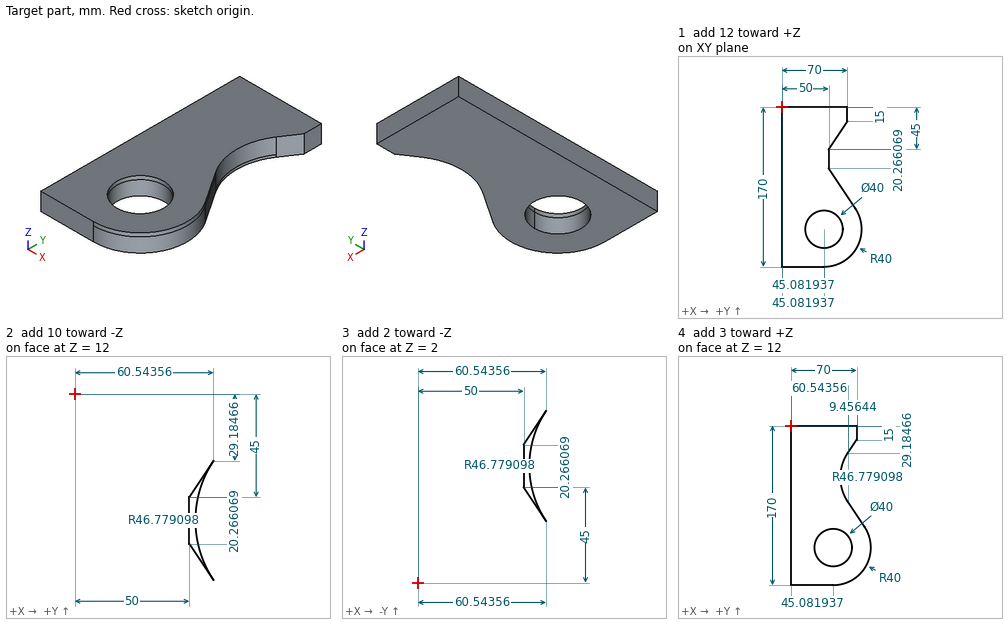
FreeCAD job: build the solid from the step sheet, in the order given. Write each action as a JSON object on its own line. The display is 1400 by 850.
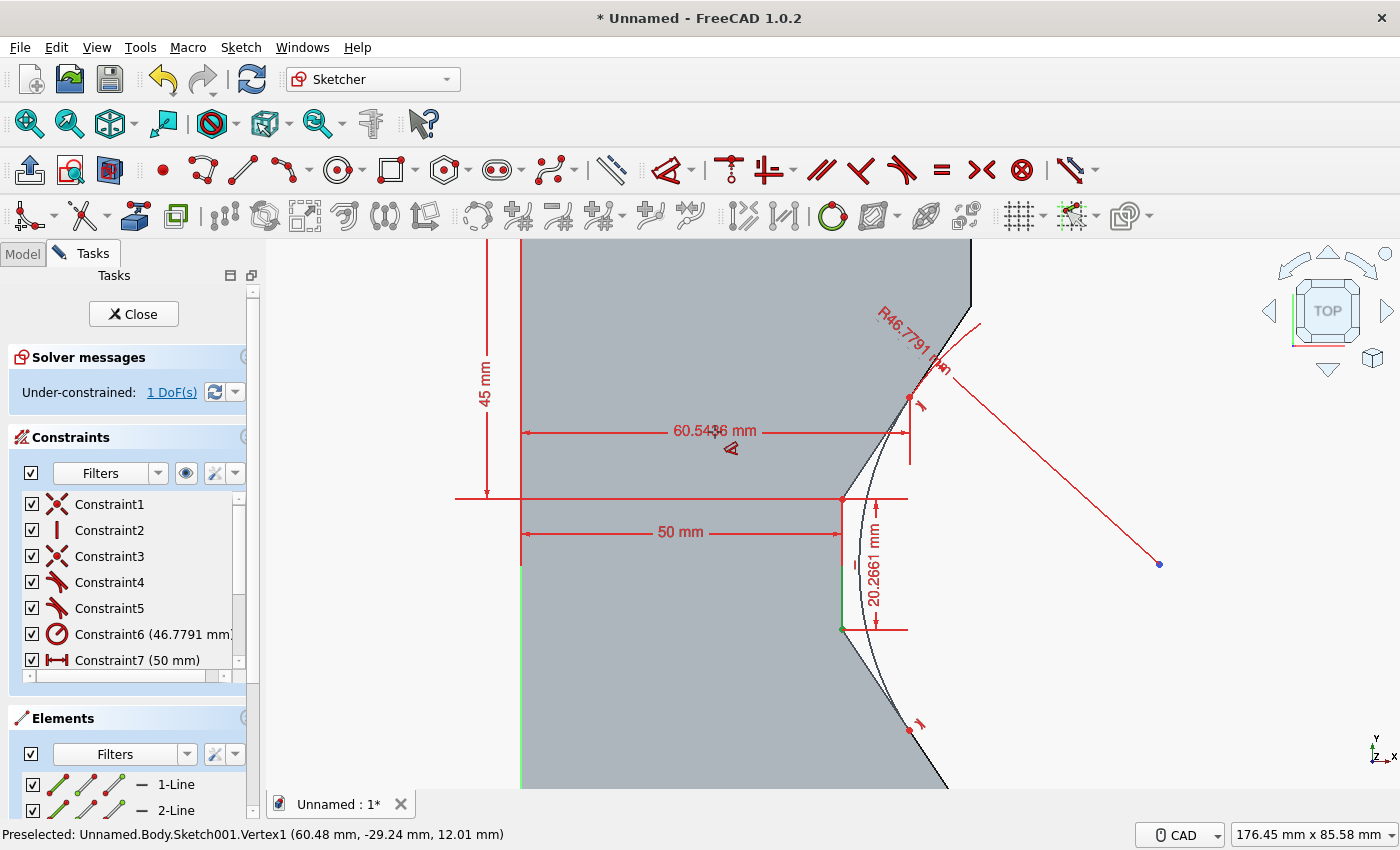
{"action": "left_click", "coordinate": [910, 398]}
{"action": "left_click", "coordinate": [487, 332]}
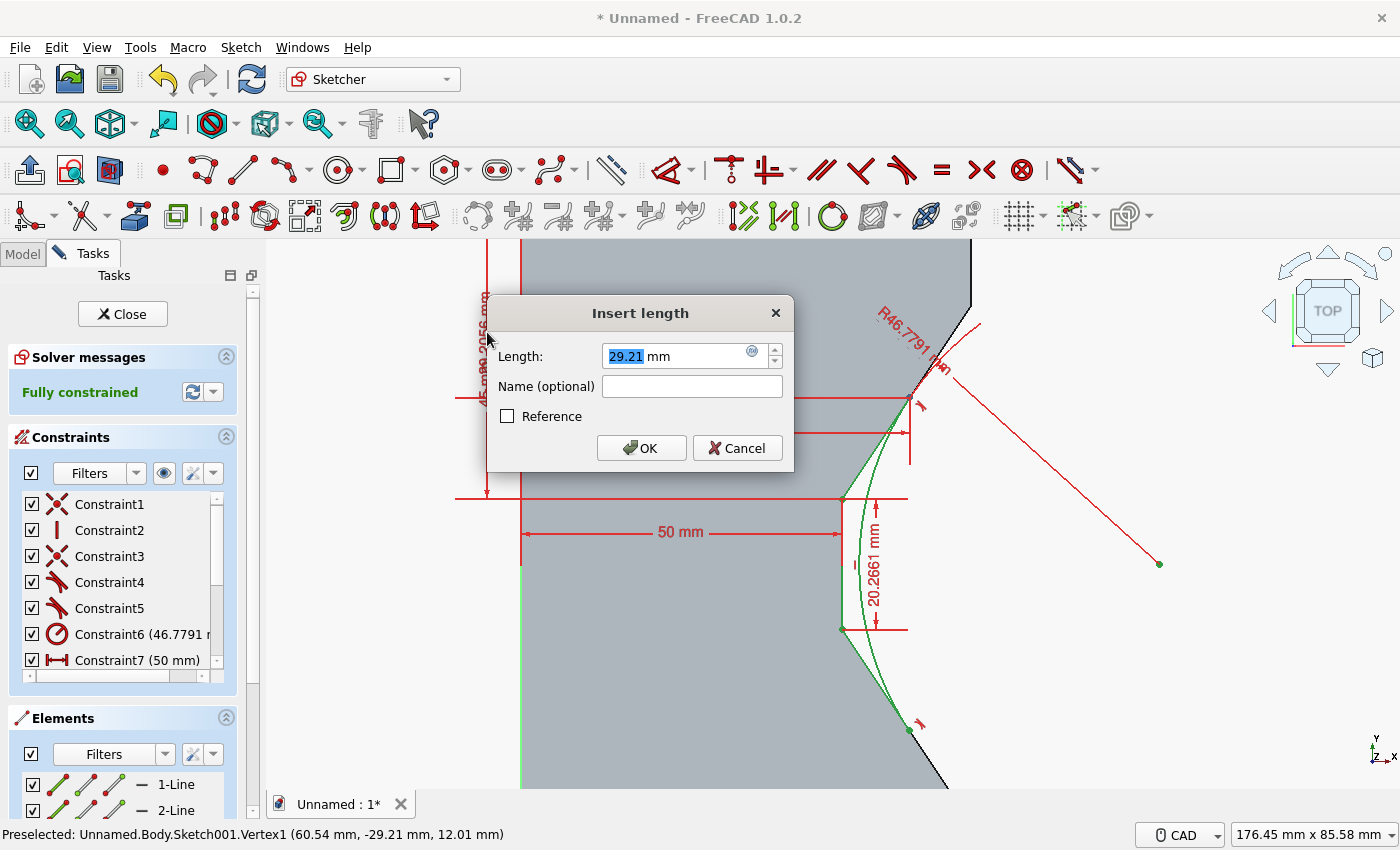
{"action": "type", "text": "29.18466"}
{"action": "key", "text": "Return"}
{"action": "key", "text": "Escape"}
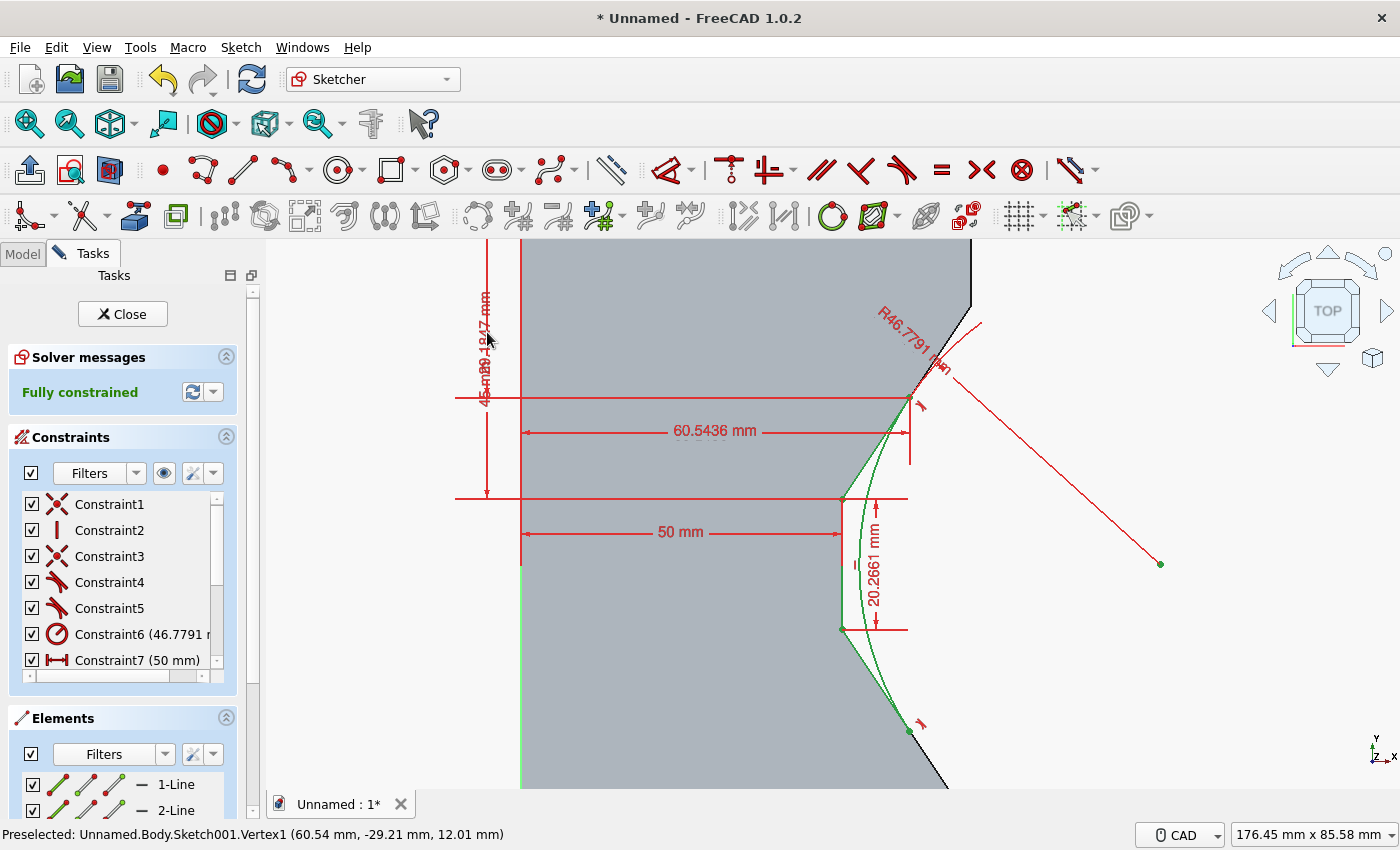
{"action": "left_click", "coordinate": [123, 314]}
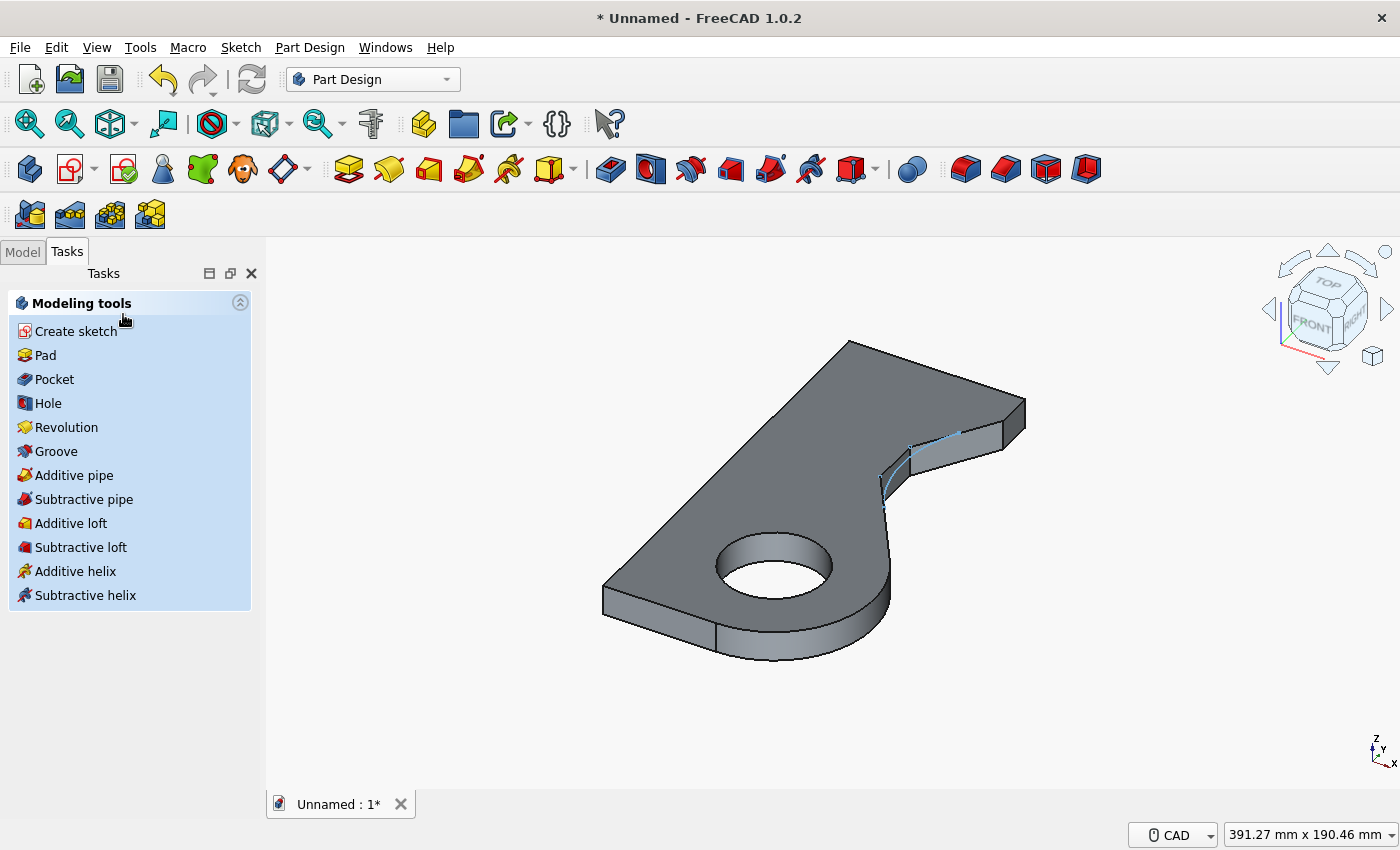
{"action": "left_click", "coordinate": [350, 170]}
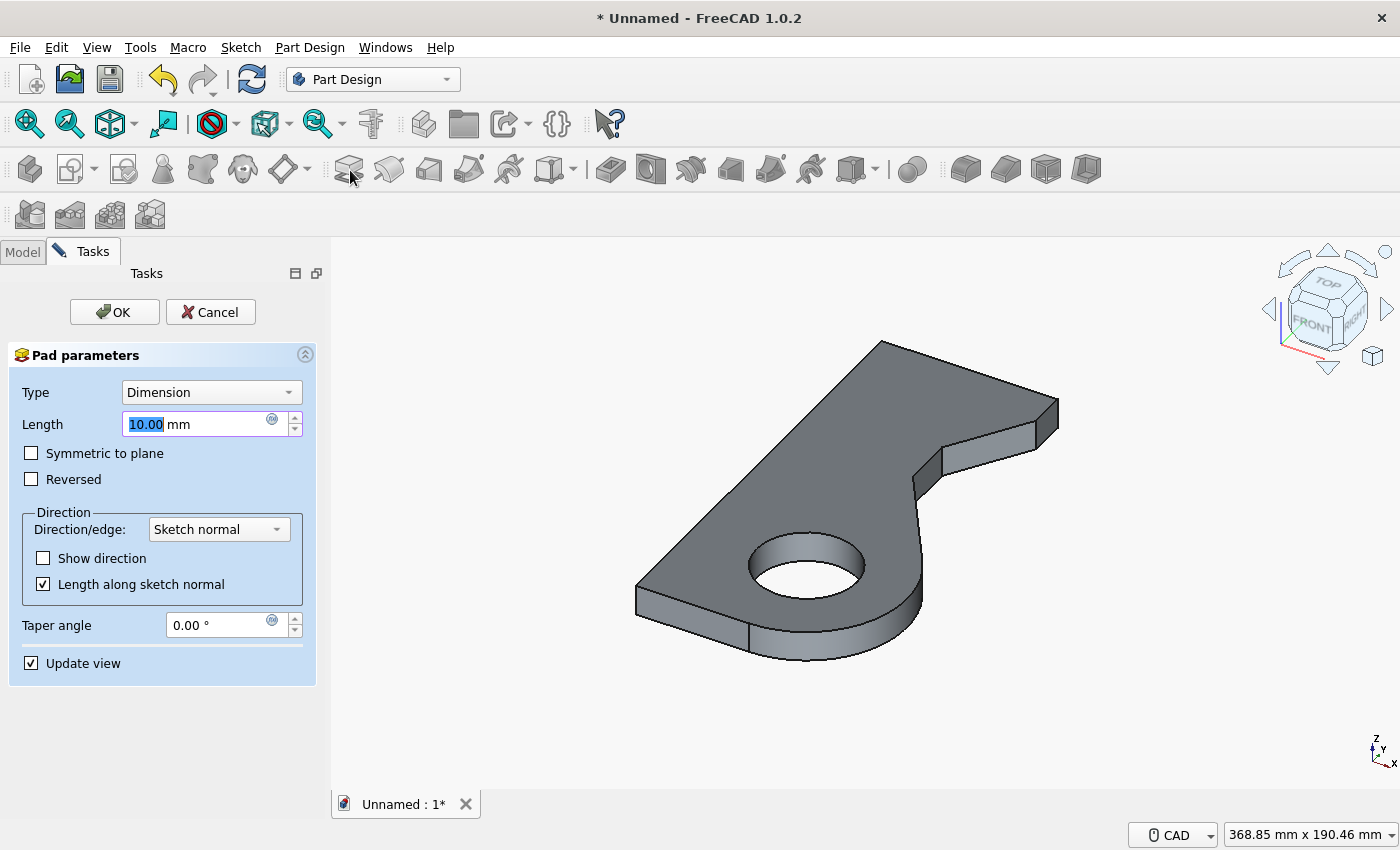
{"action": "type", "text": "10"}
{"action": "key", "text": "Tab"}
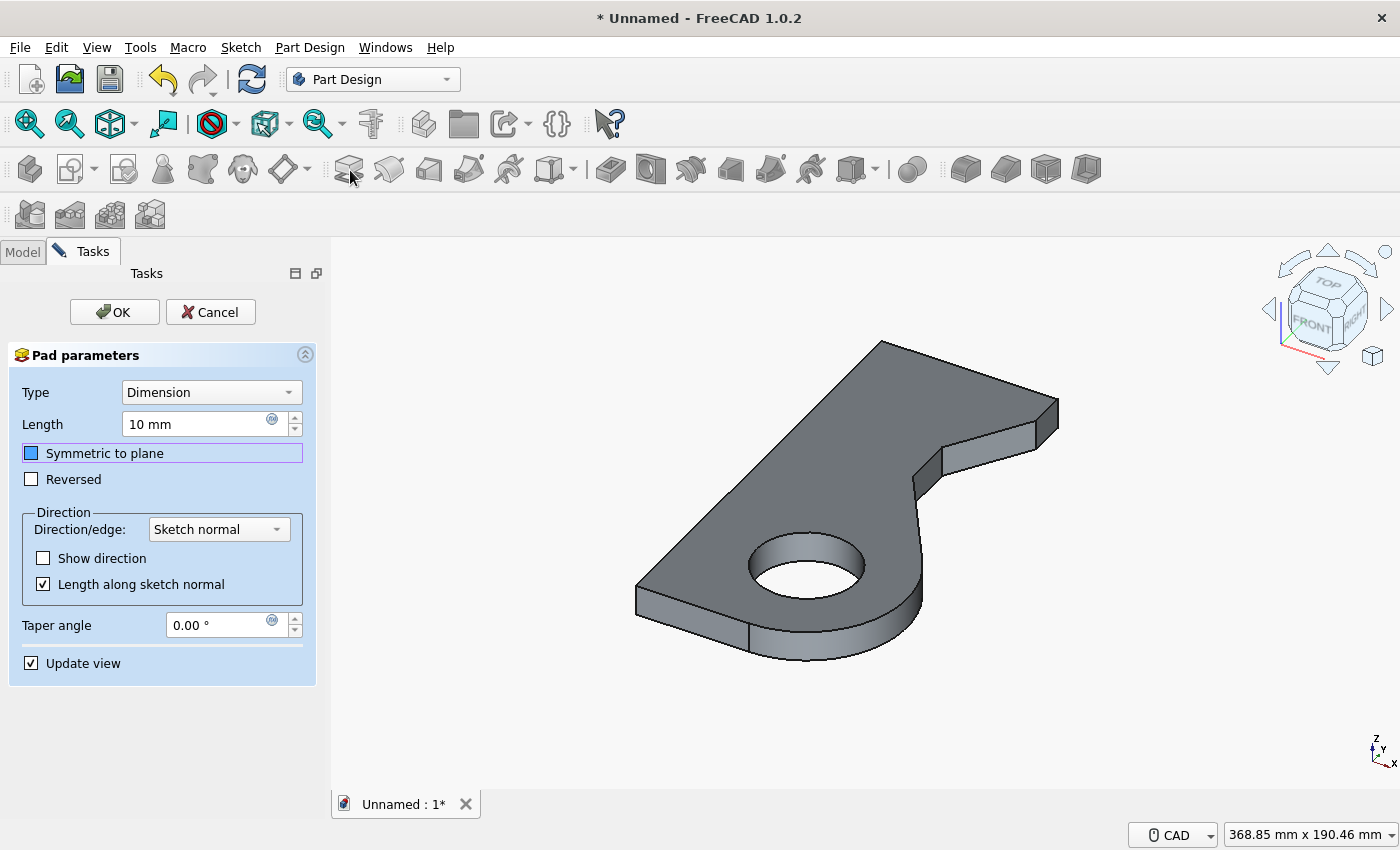
{"action": "left_click", "coordinate": [30, 479]}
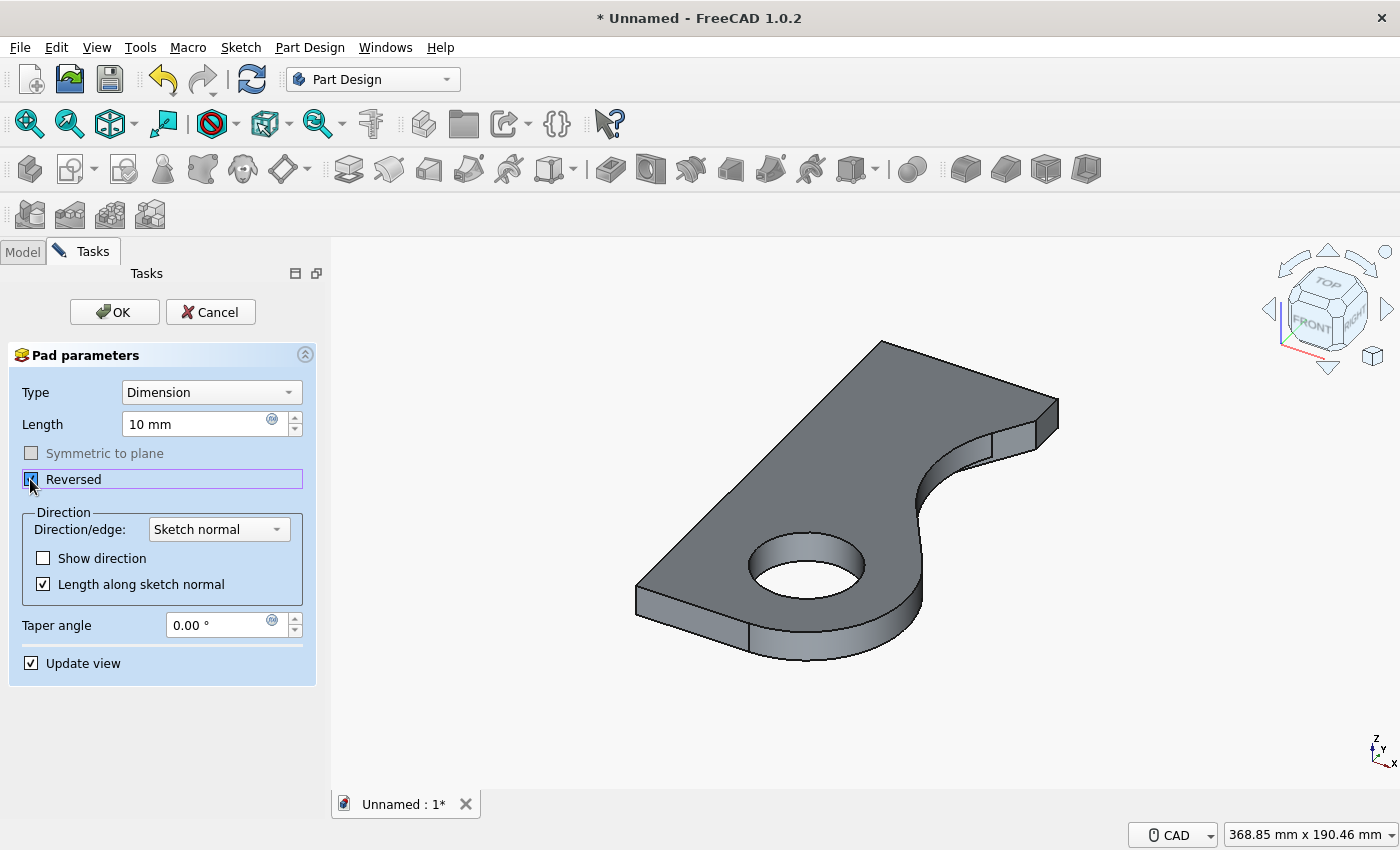
{"action": "left_click", "coordinate": [115, 312]}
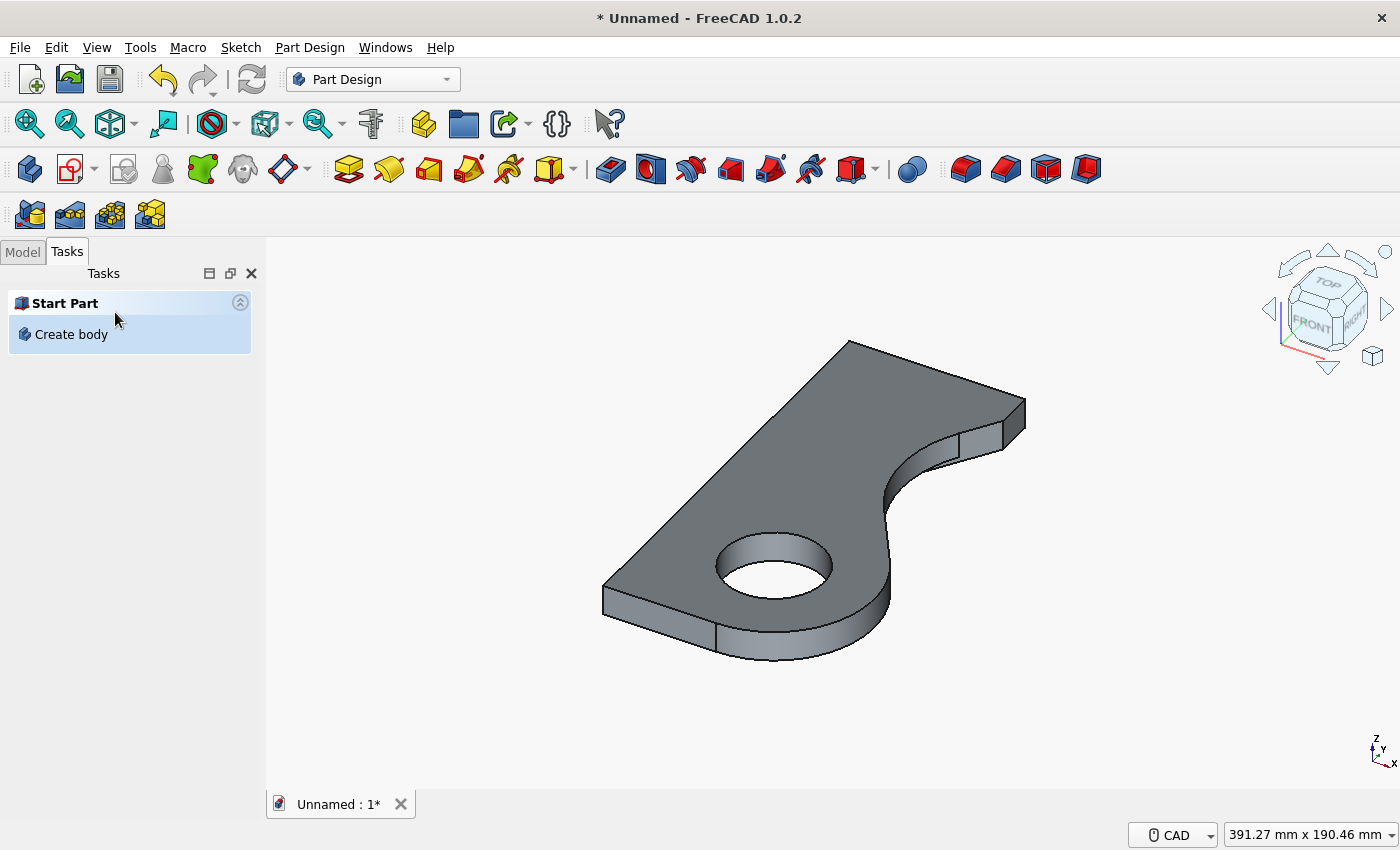
{"action": "key", "text": "5"}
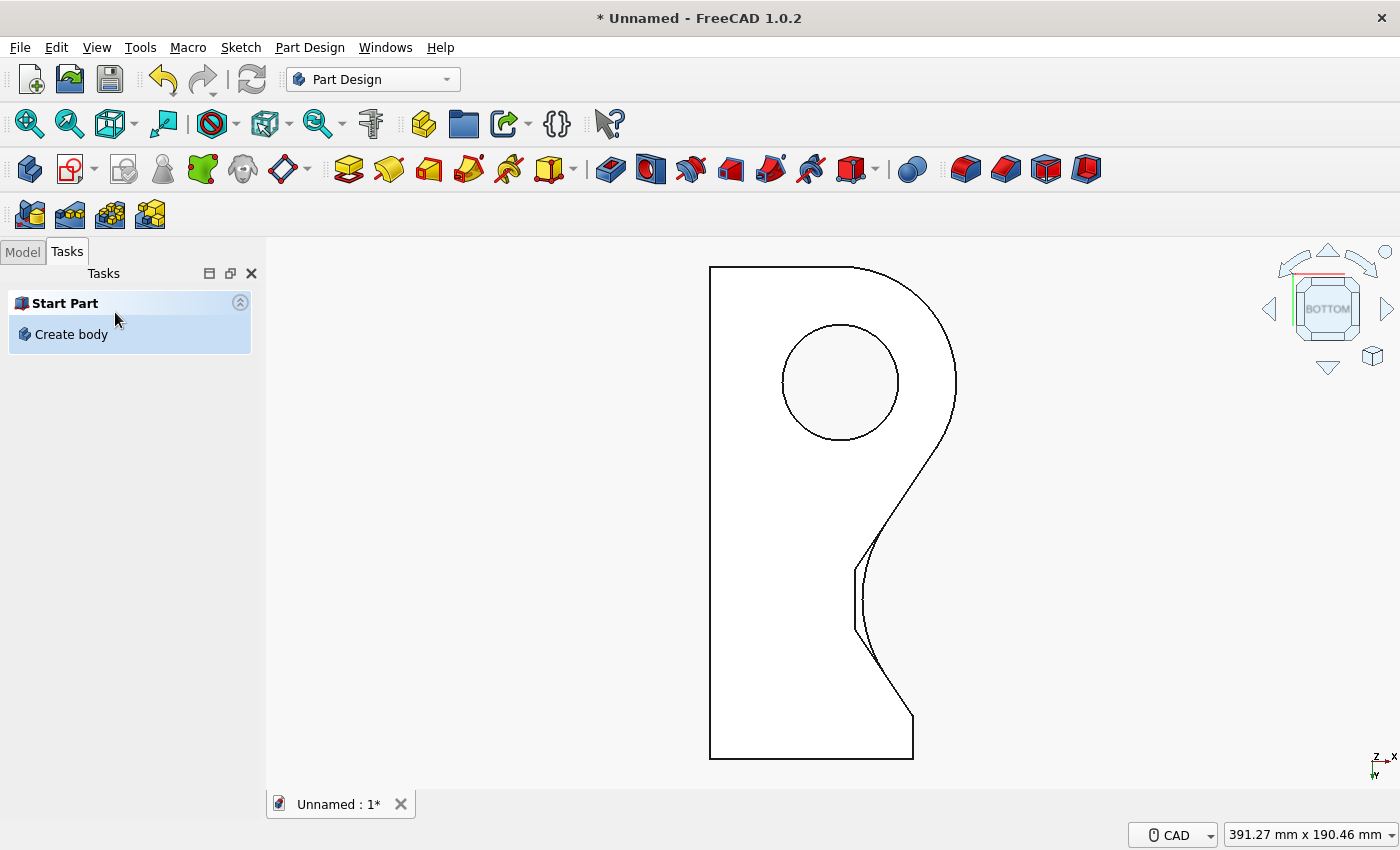
{"action": "scroll", "coordinate": [861, 620], "scroll_direction": "up", "scroll_amount": 8}